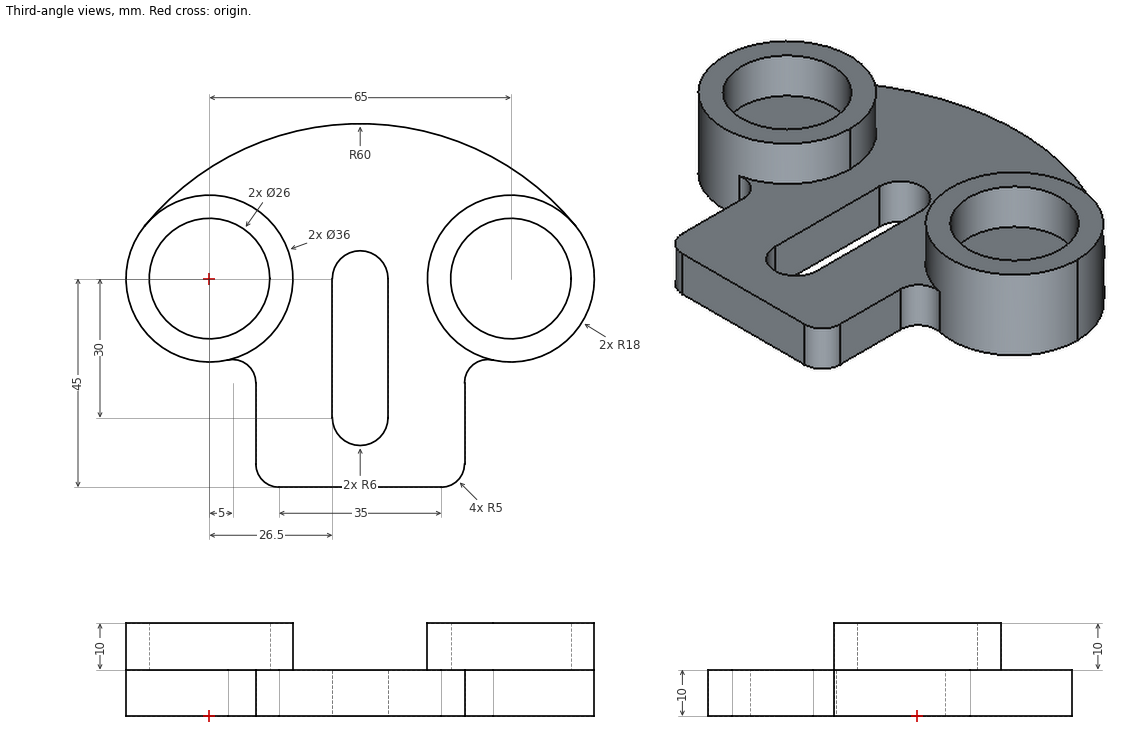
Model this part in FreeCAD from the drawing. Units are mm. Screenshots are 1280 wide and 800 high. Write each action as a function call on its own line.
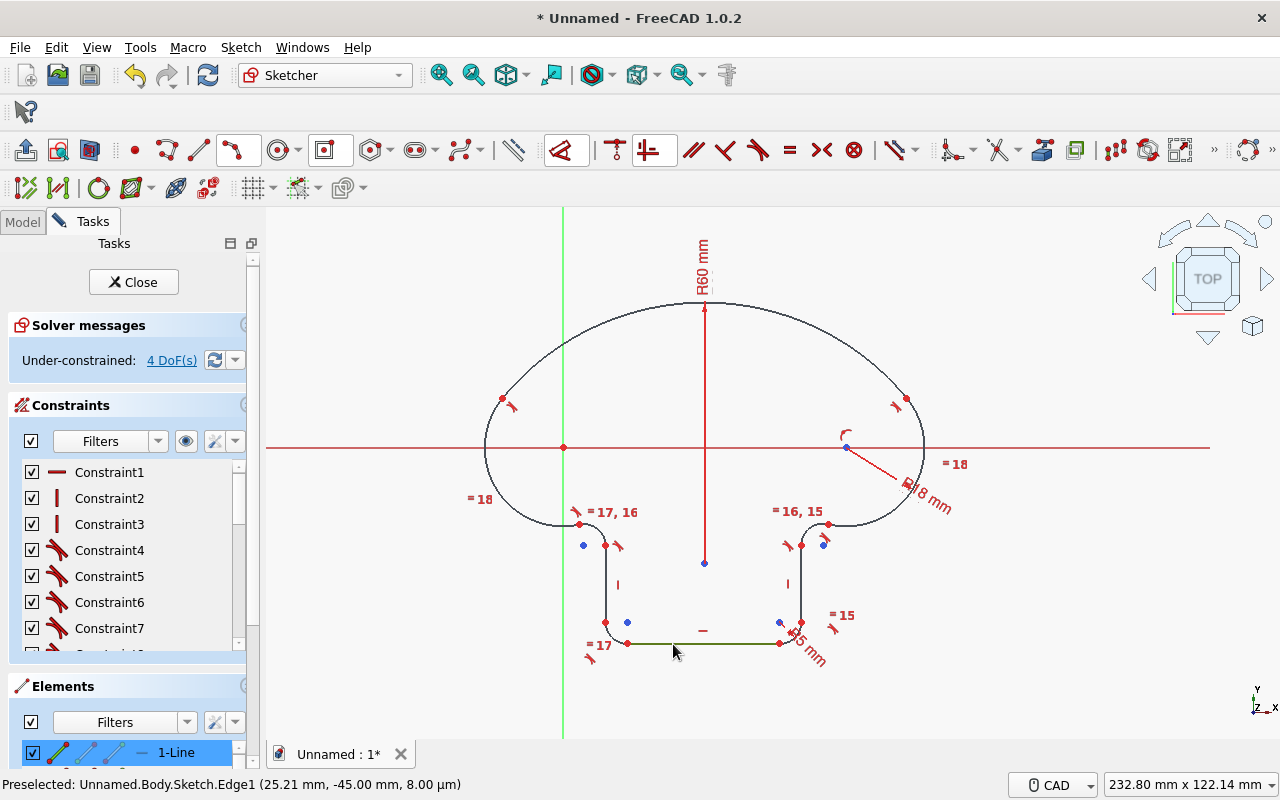
click(584, 150)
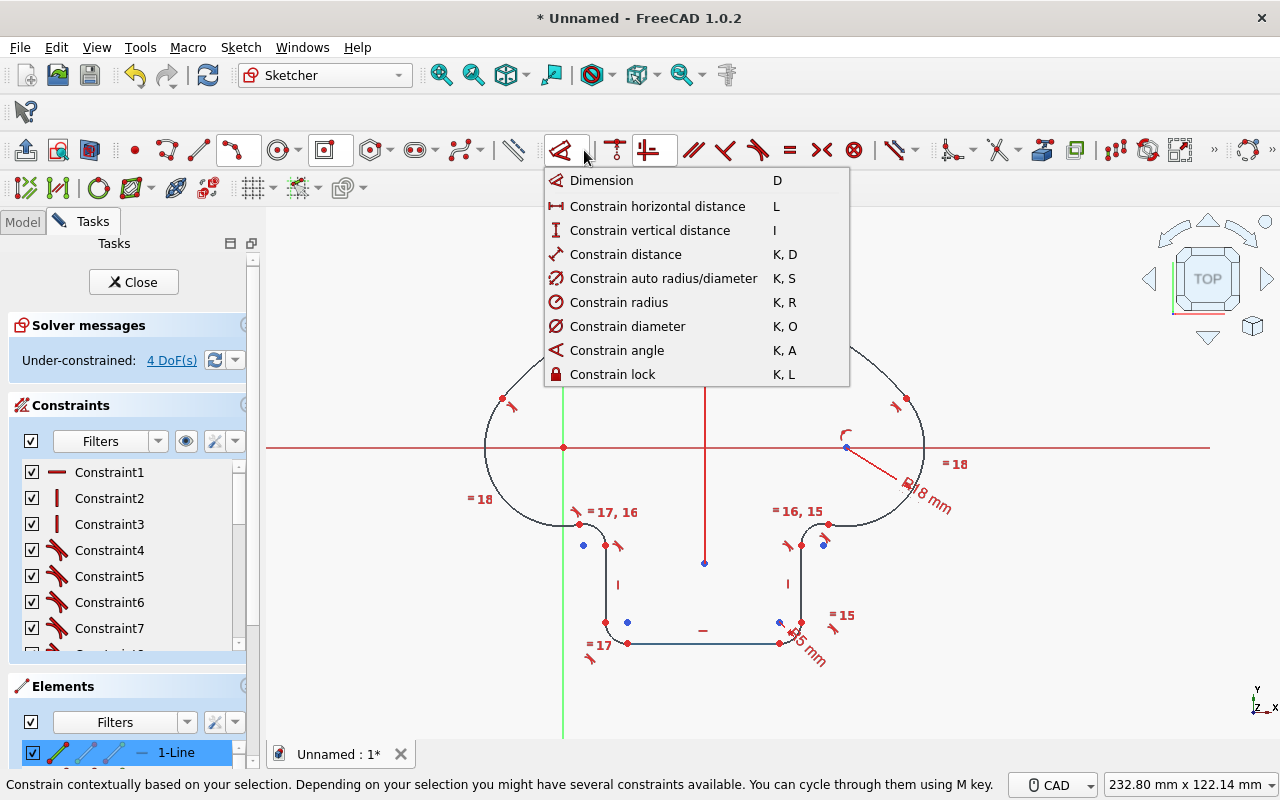
click(697, 206)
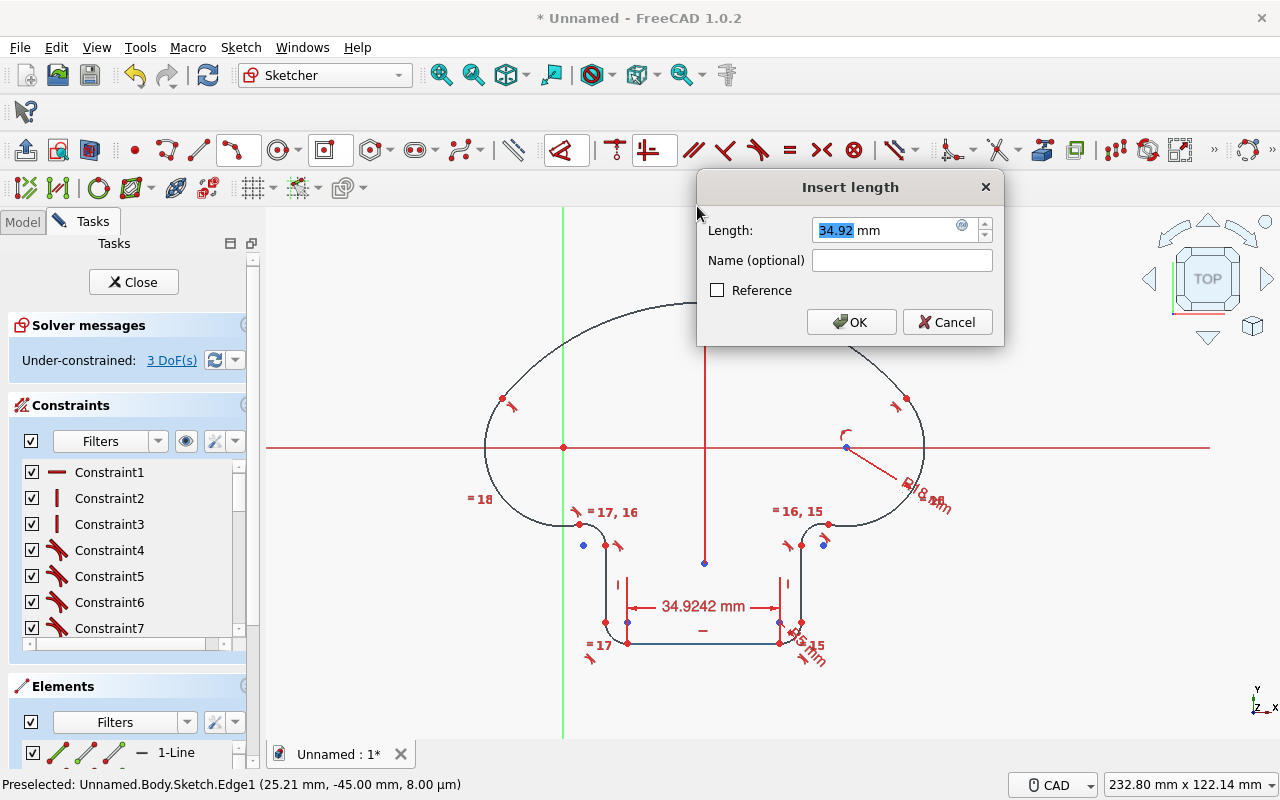
text(35)
key(Return)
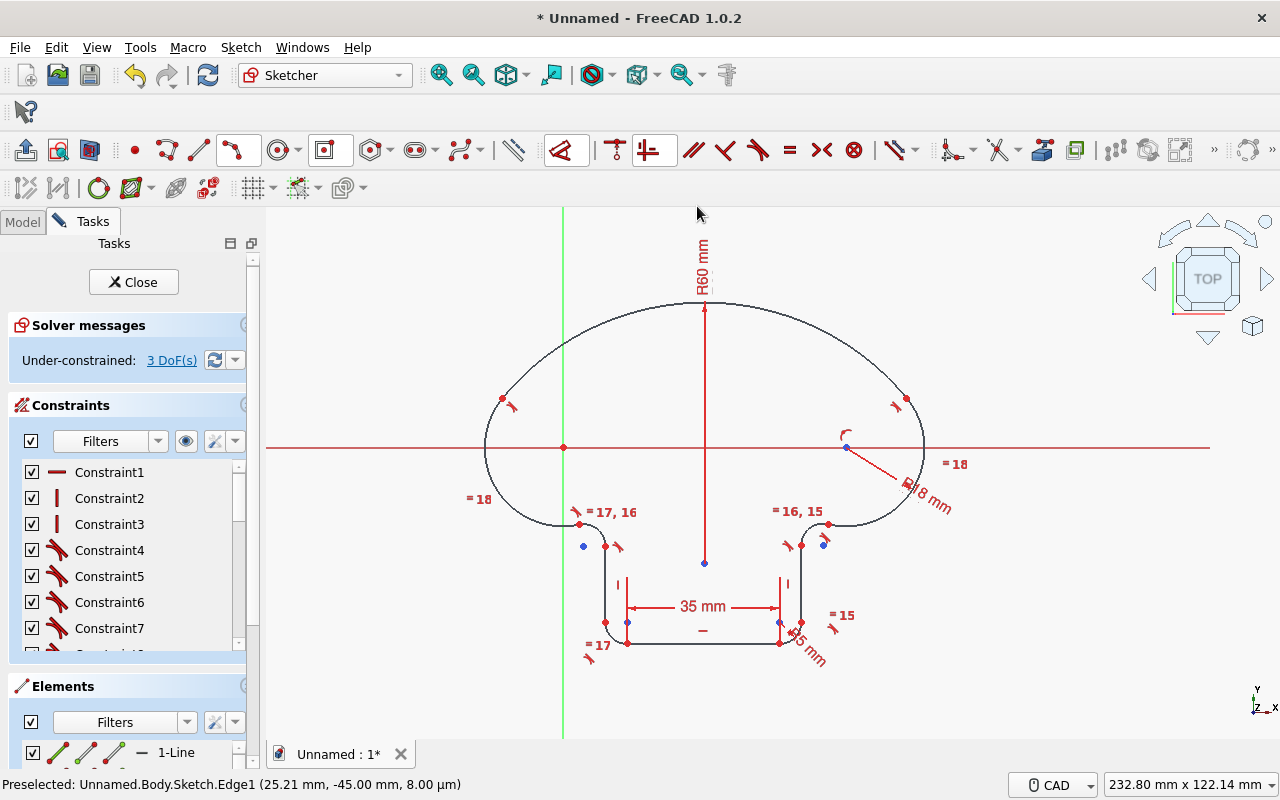
scroll(584, 546, up, 4)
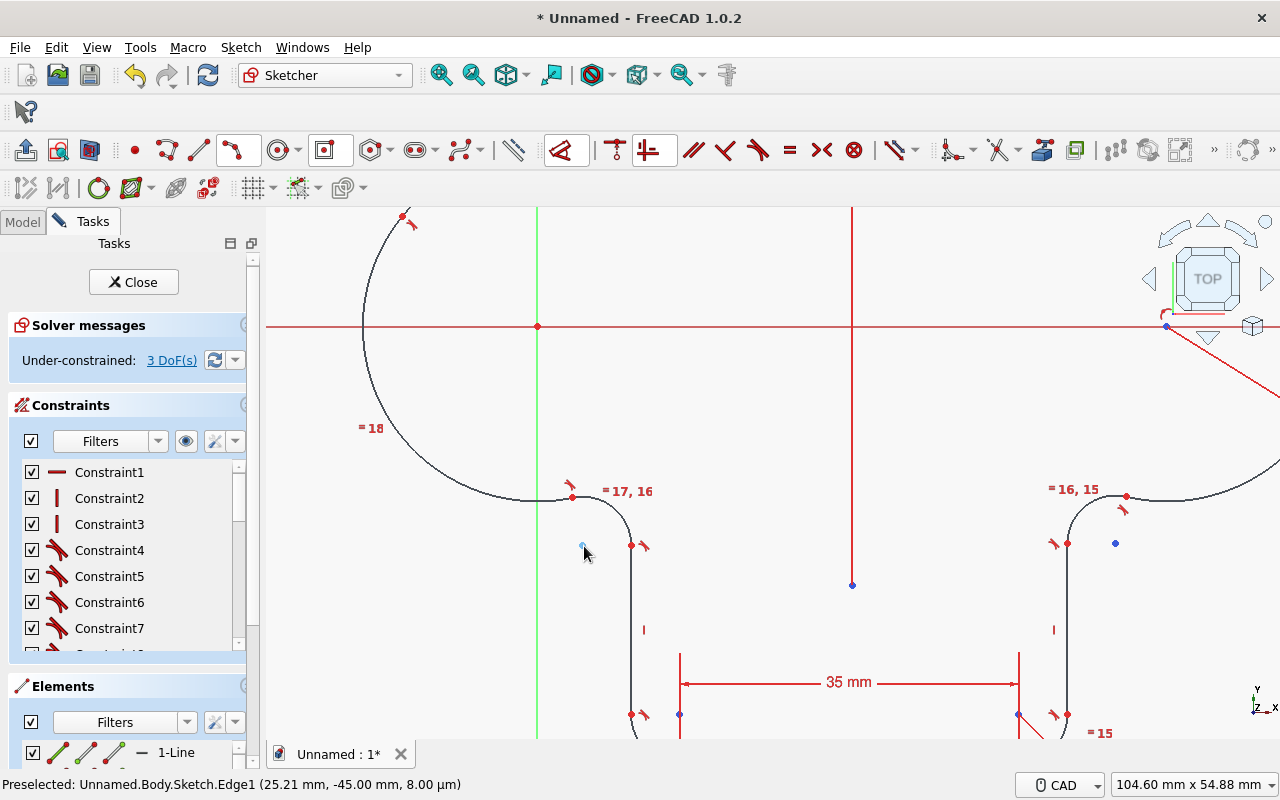
click(583, 545)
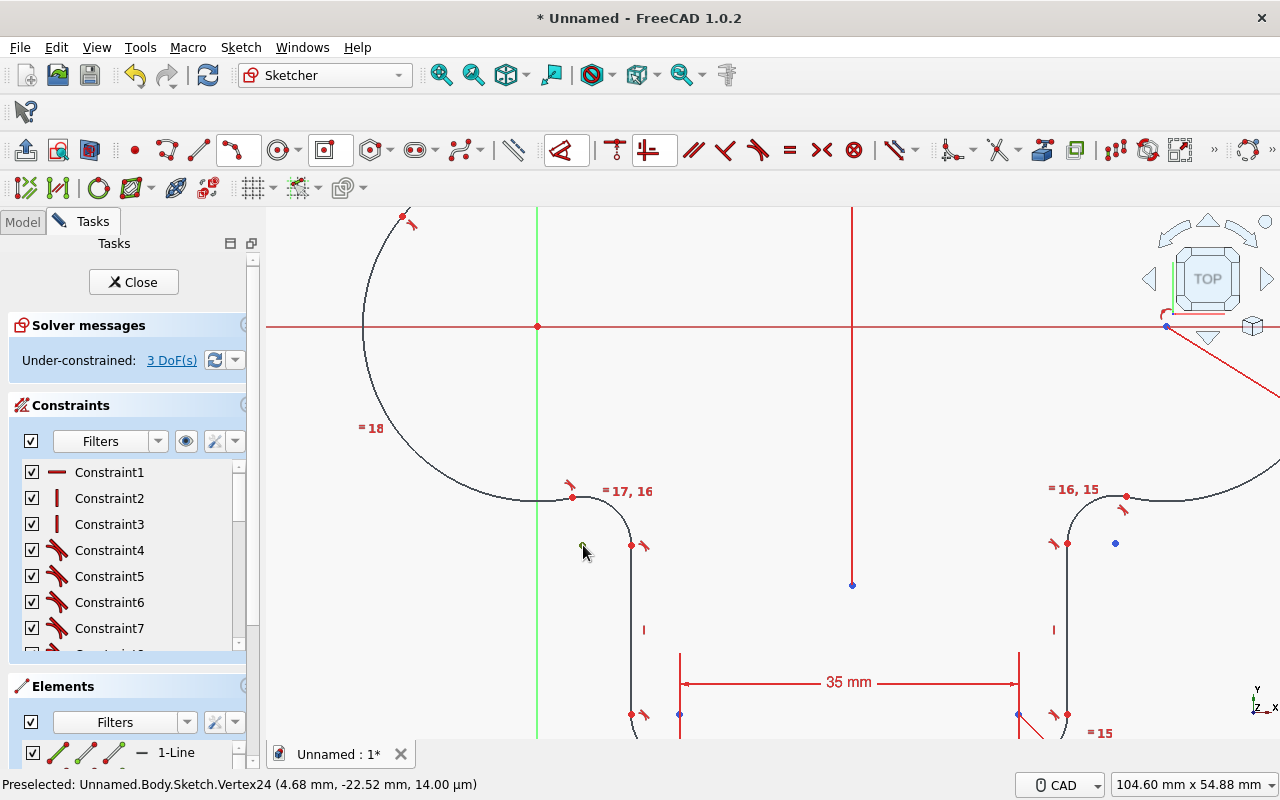
click(584, 150)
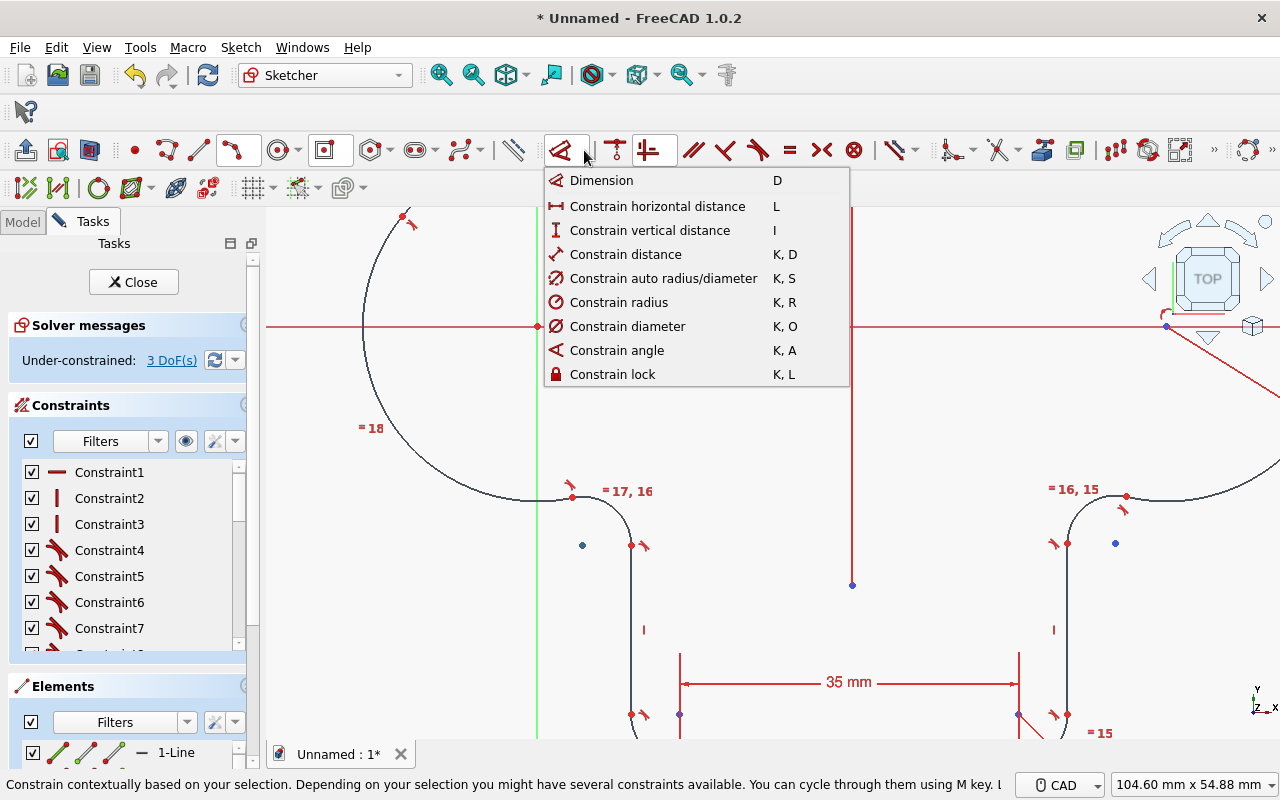
click(697, 206)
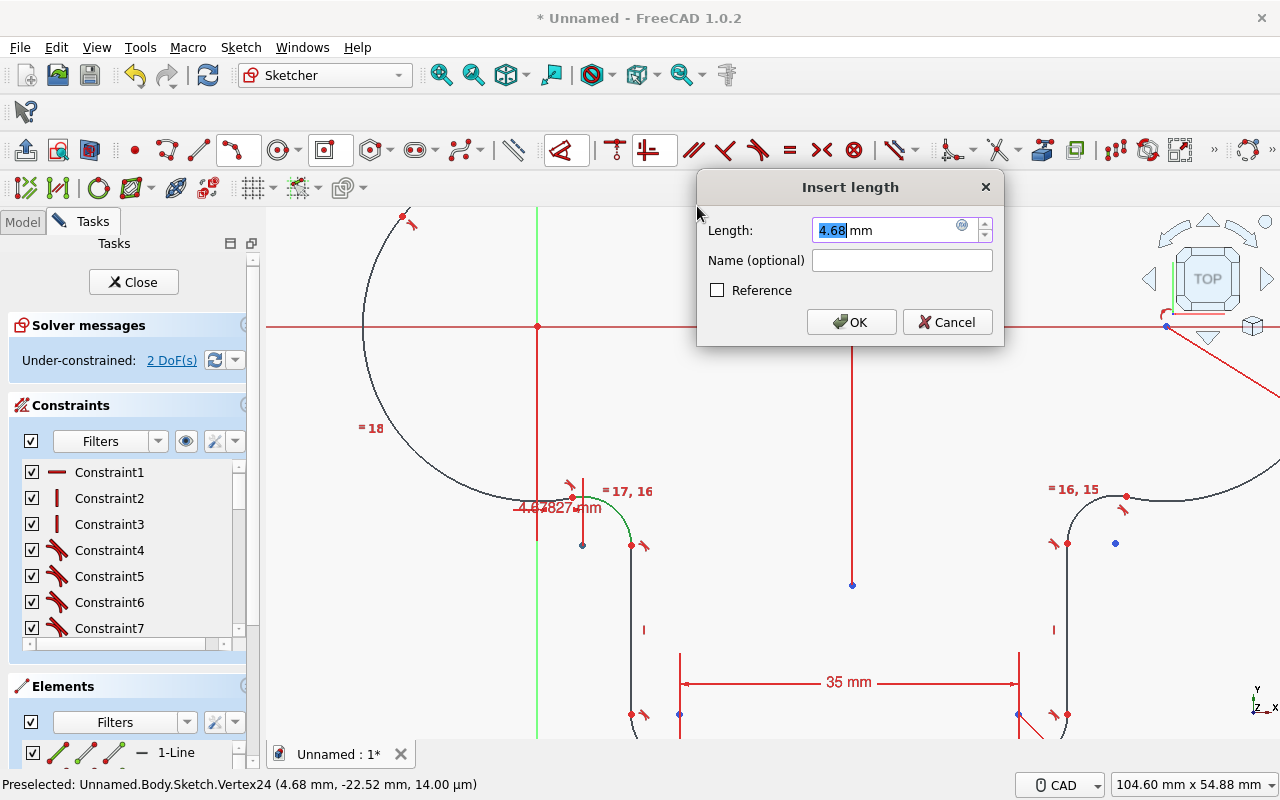
text(5)
key(Return)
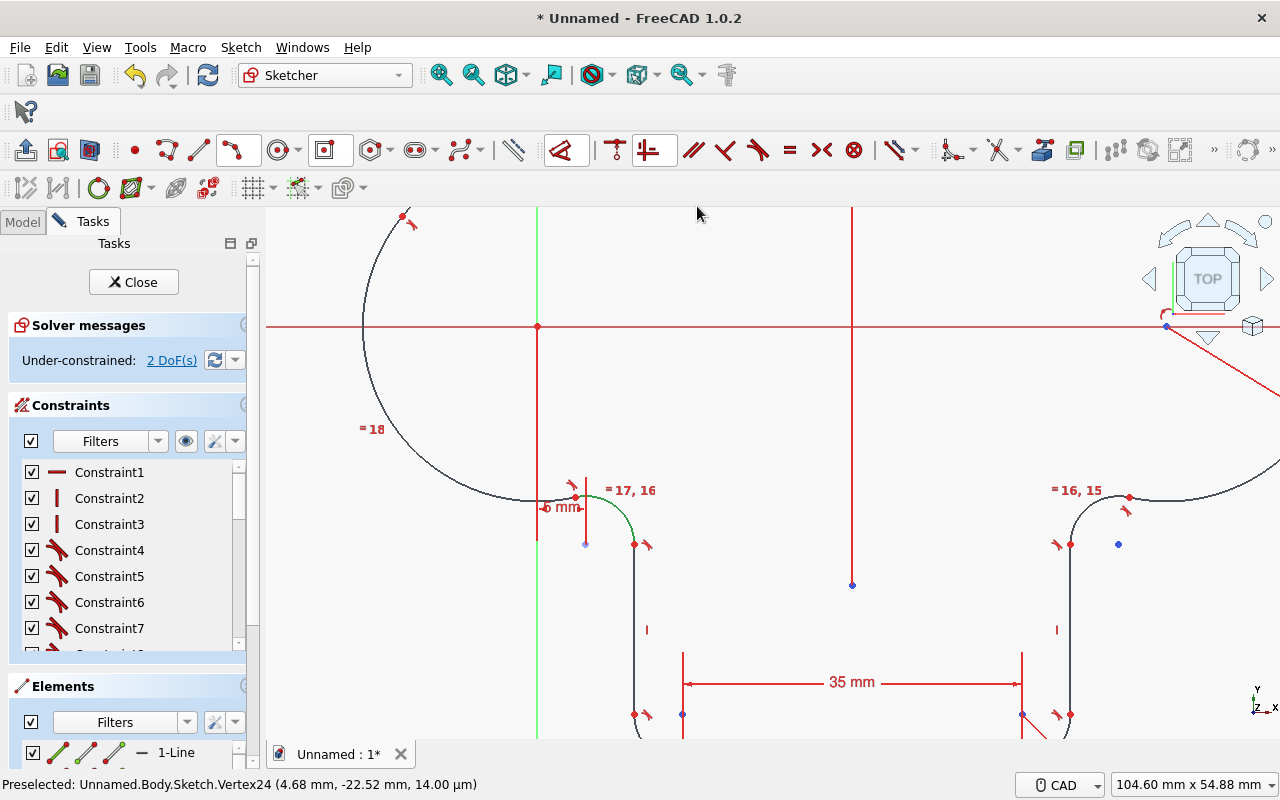
scroll(584, 546, down, 4)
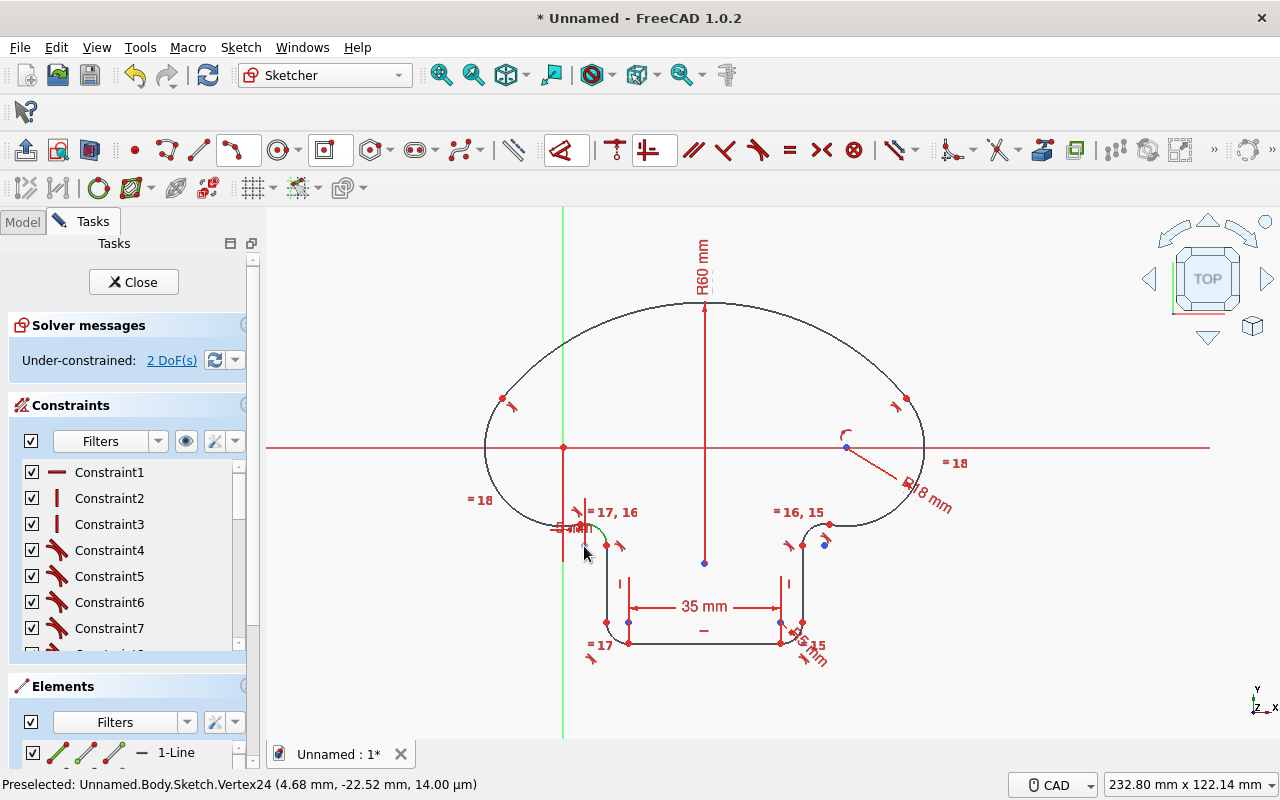
click(629, 644)